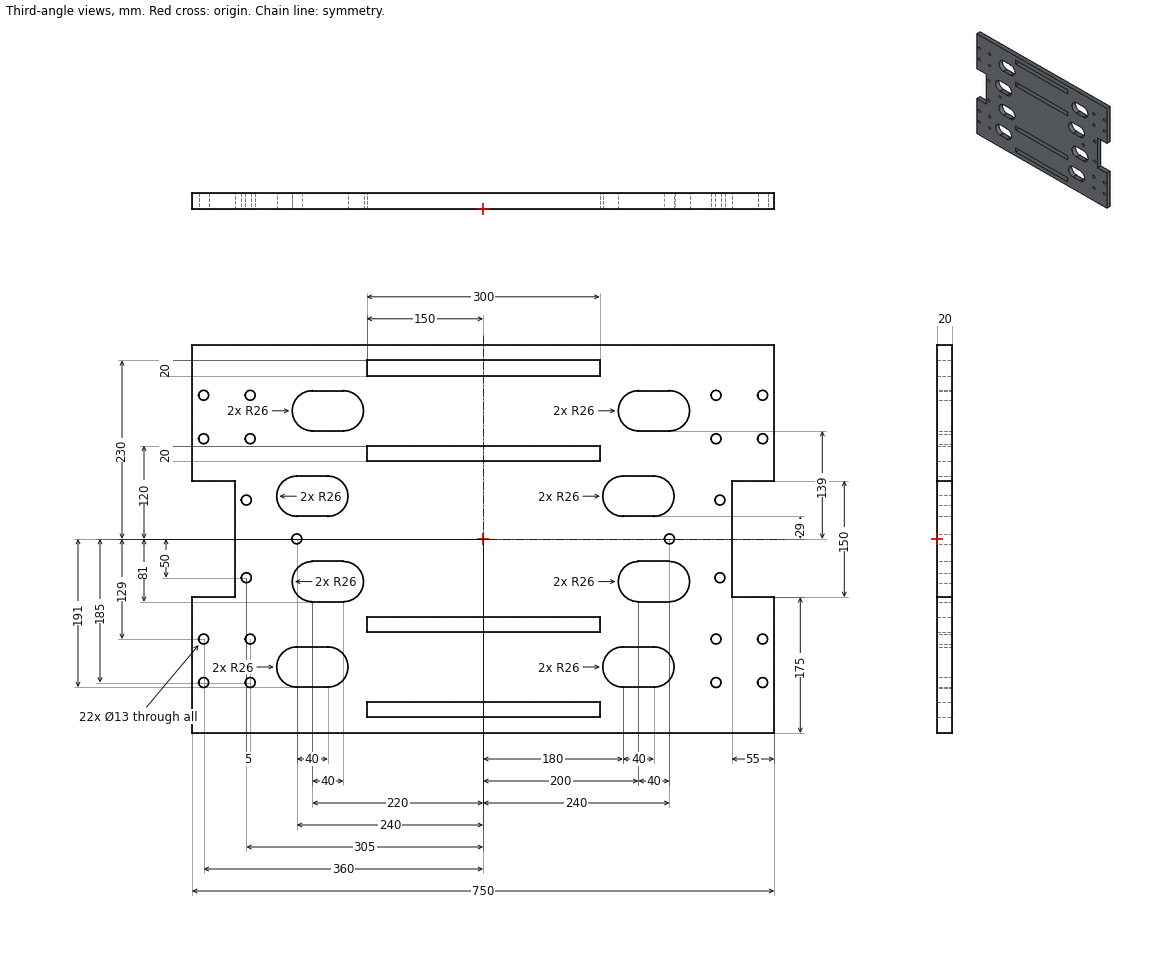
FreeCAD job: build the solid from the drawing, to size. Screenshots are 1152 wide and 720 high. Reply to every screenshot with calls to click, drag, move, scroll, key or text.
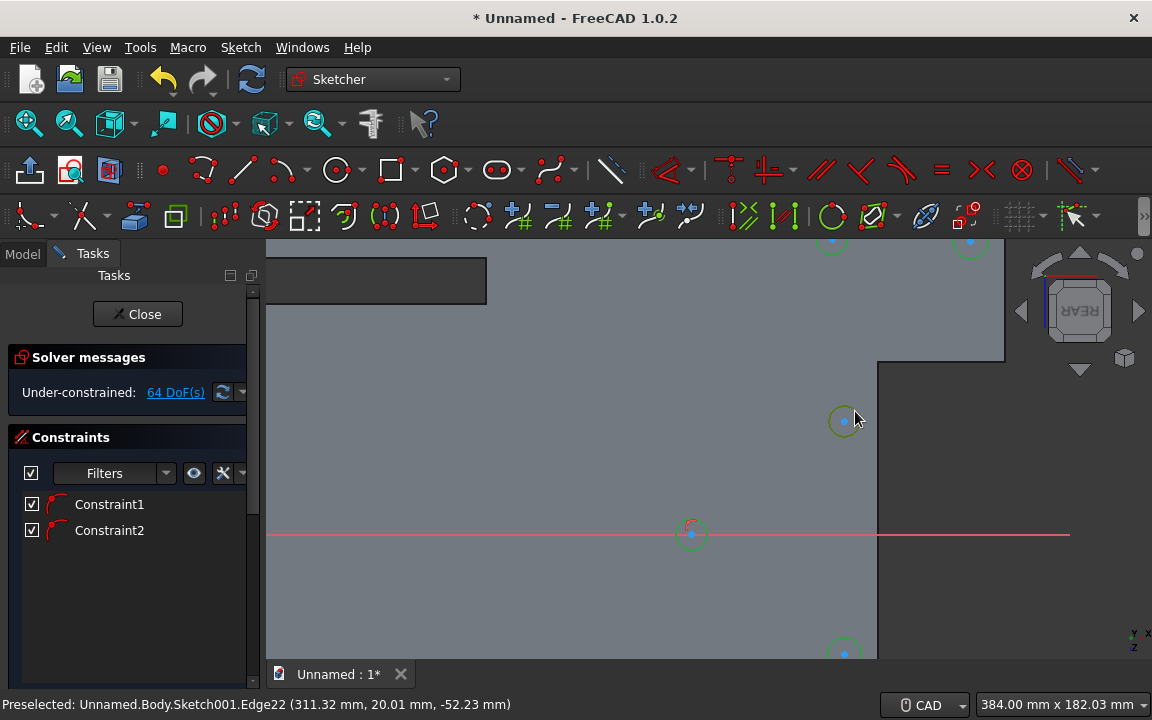
click(942, 170)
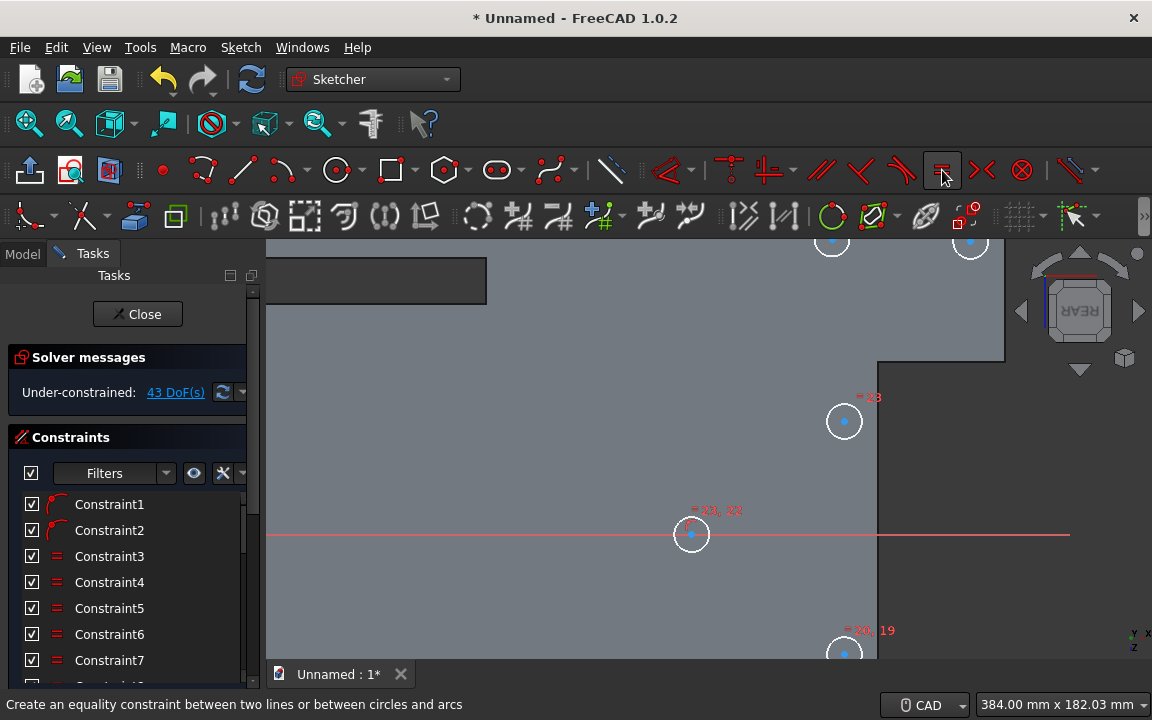
scroll(856, 412, down, 6)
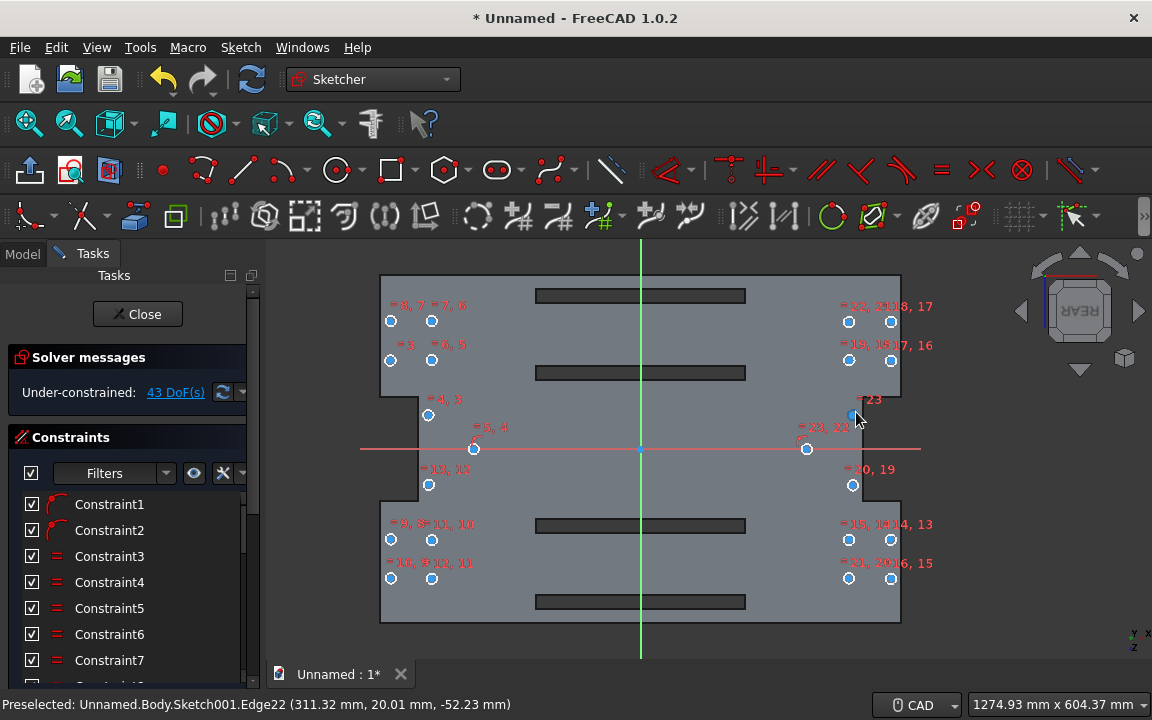
click(390, 361)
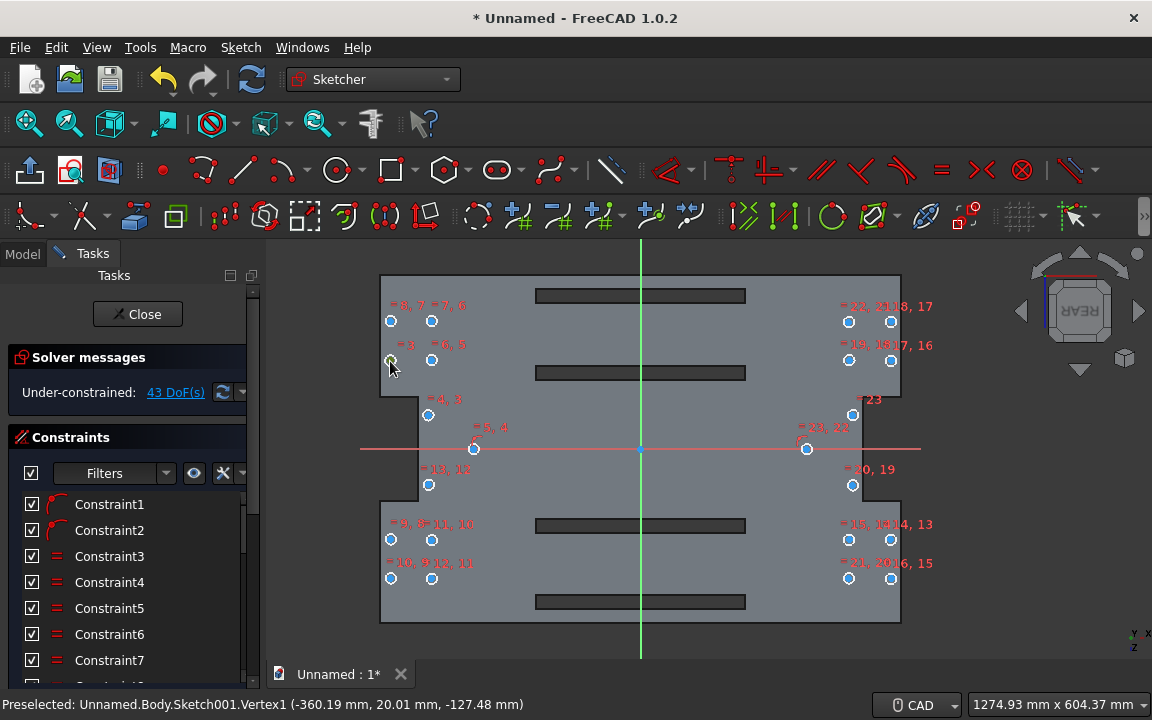
click(391, 539)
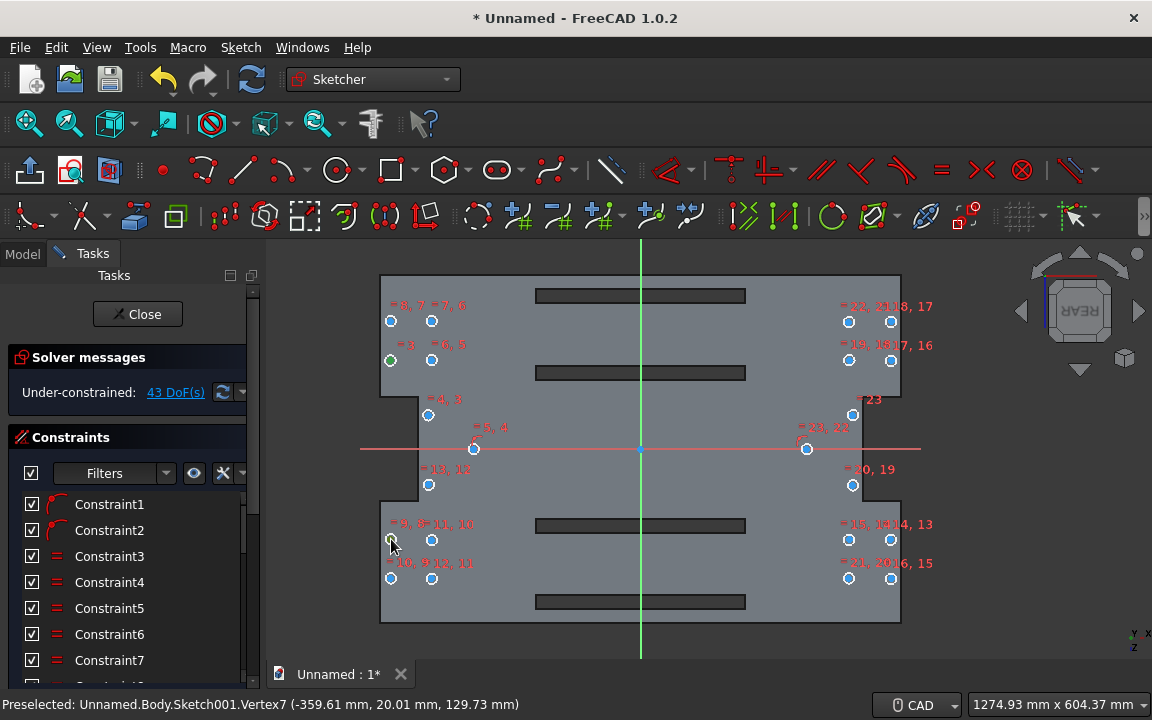
click(393, 449)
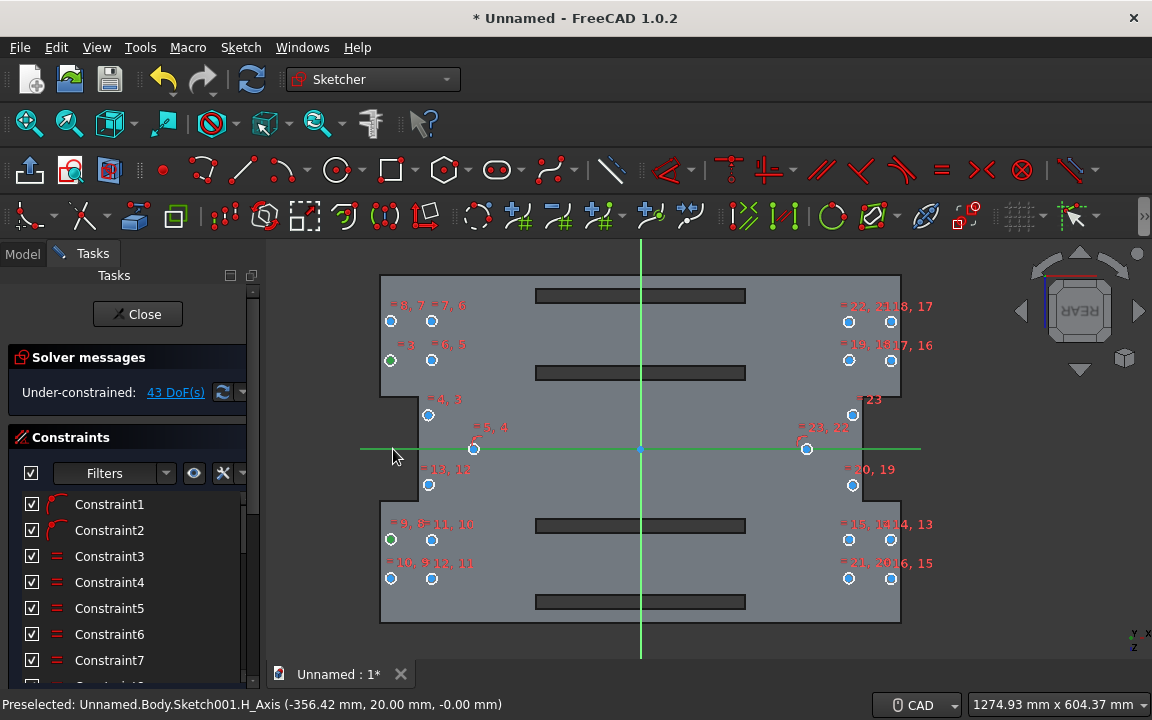
click(982, 170)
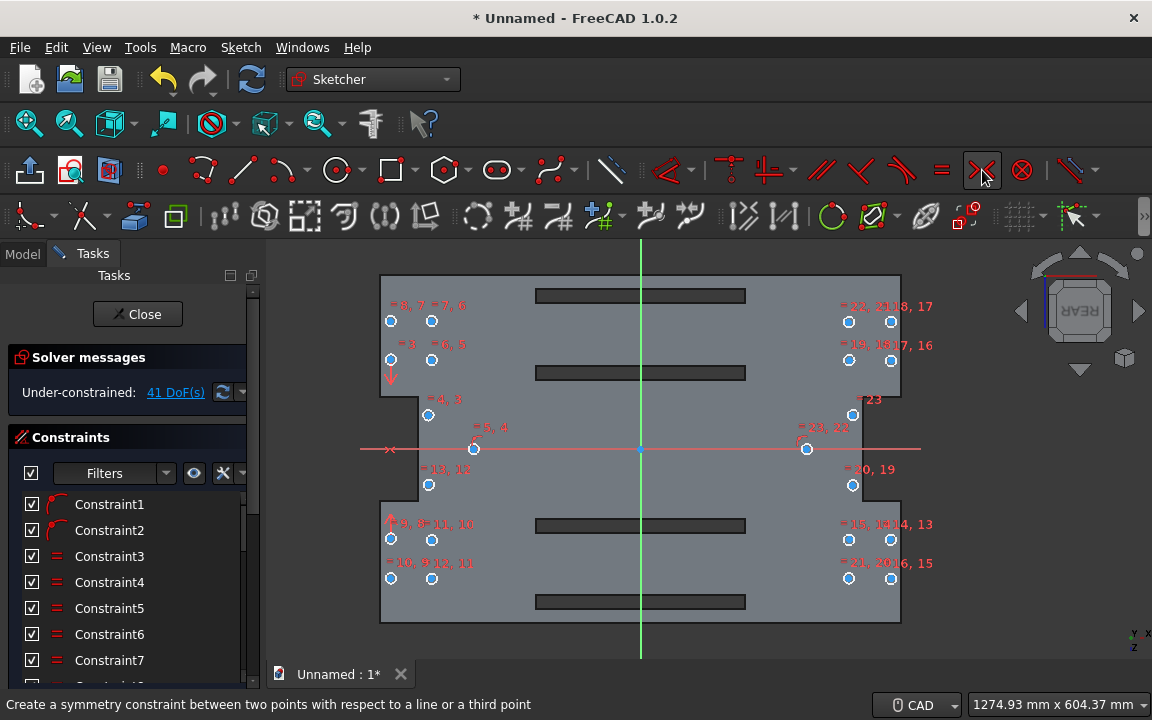
click(391, 321)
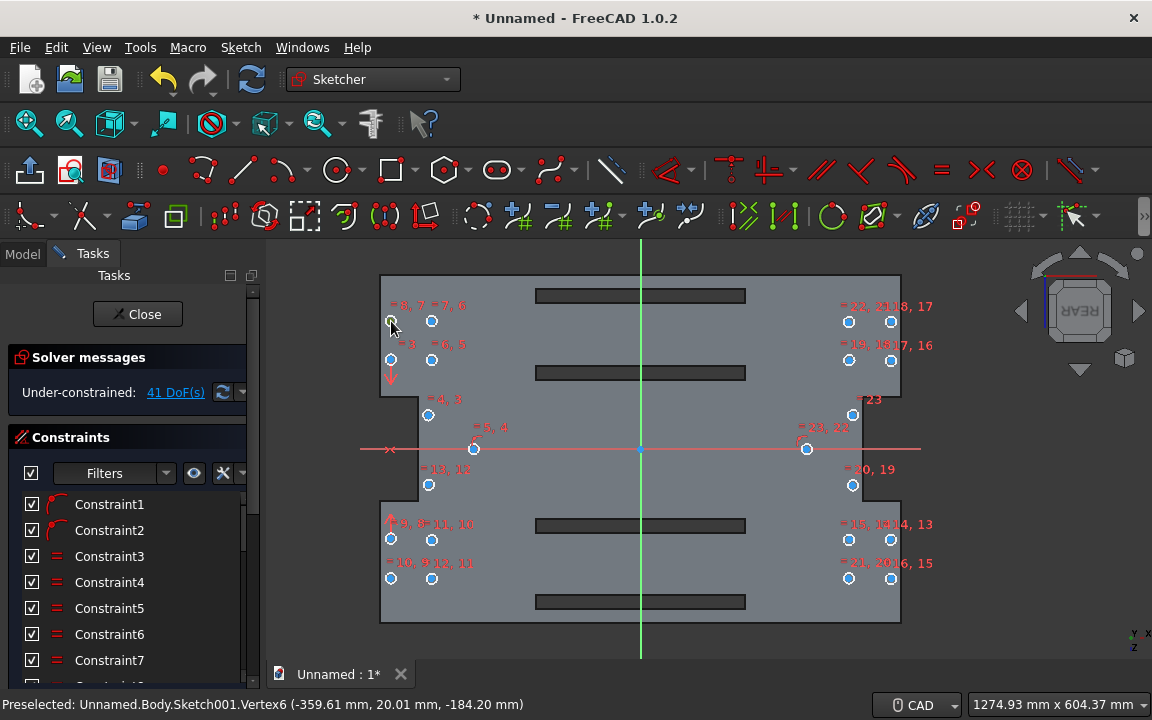
click(391, 578)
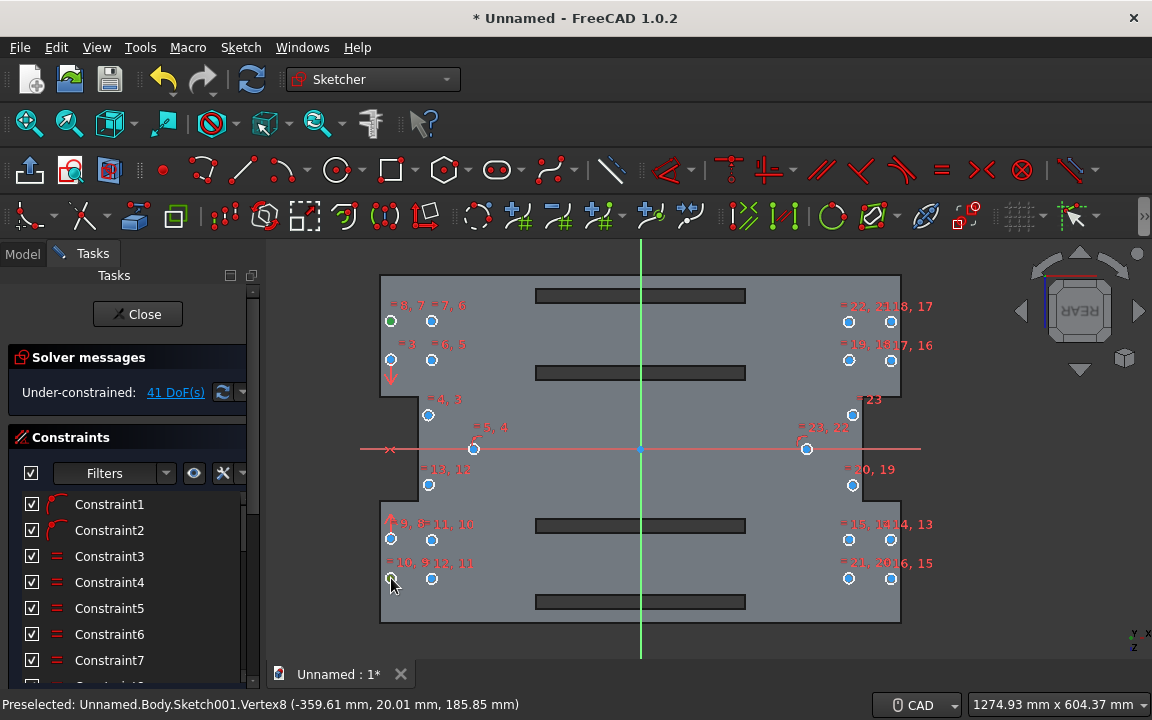
click(542, 449)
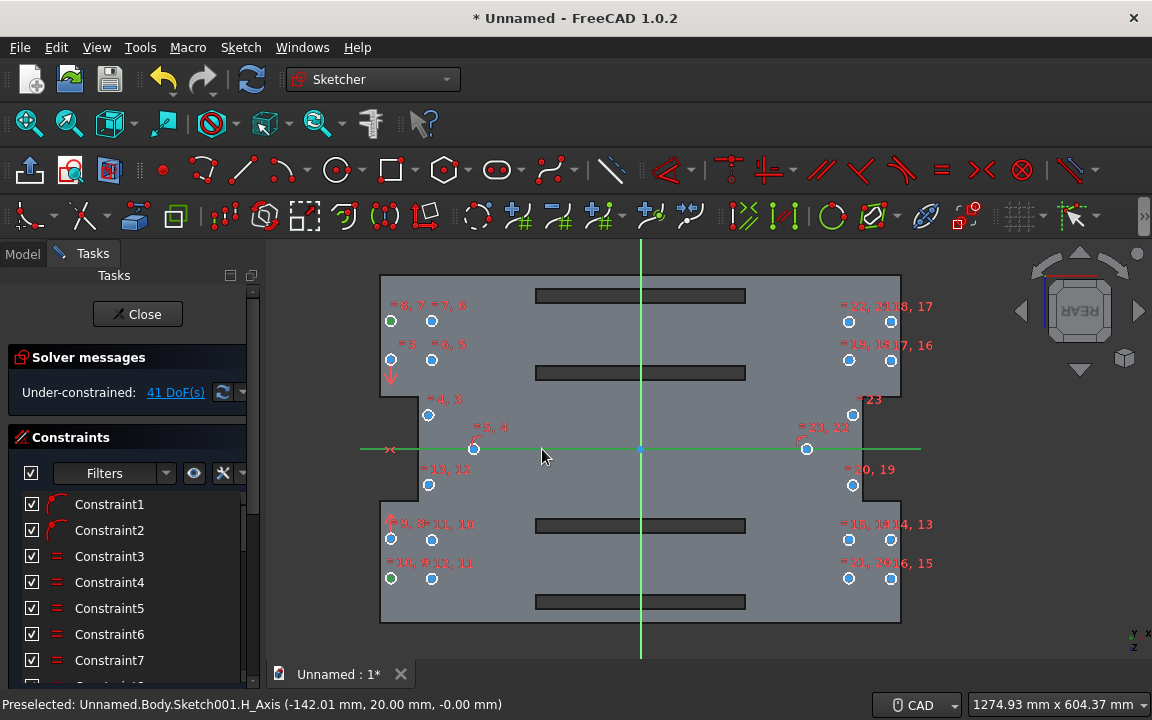
click(982, 170)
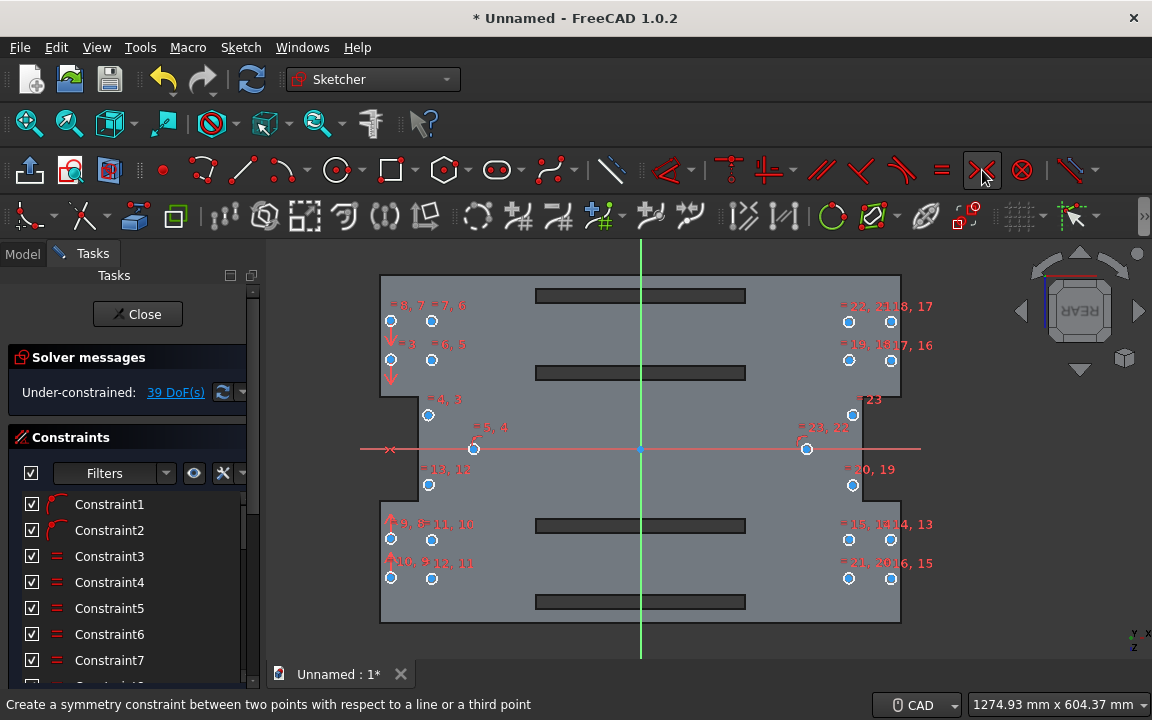
click(432, 360)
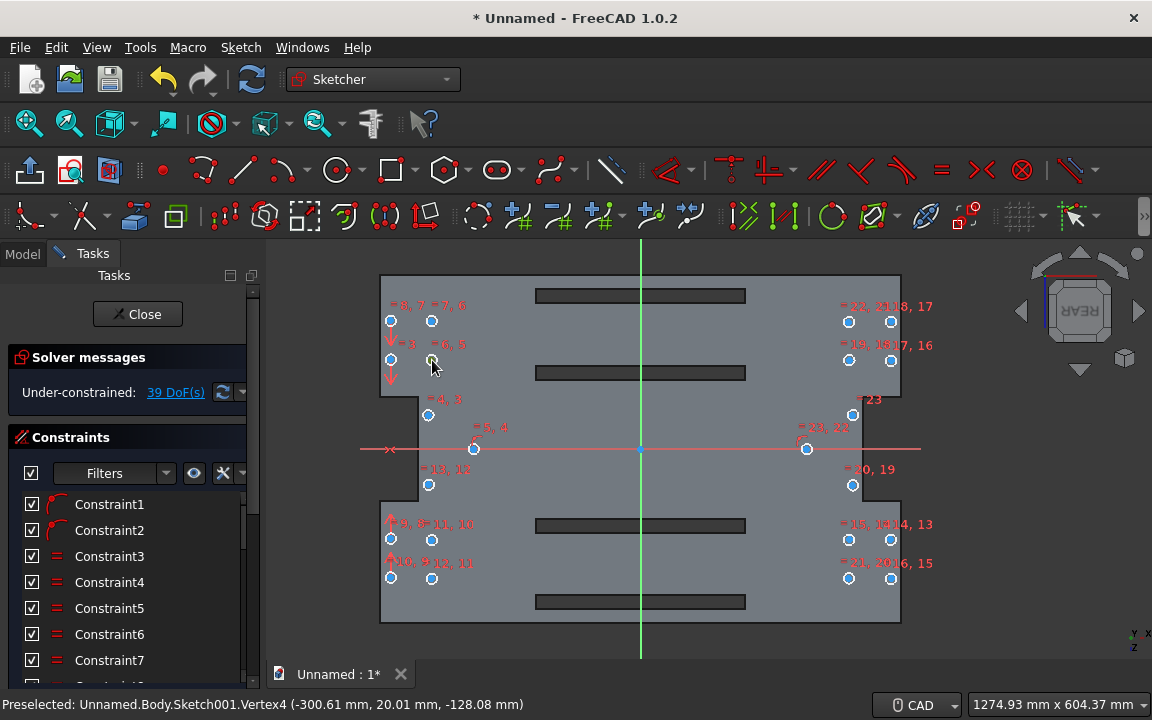
click(432, 540)